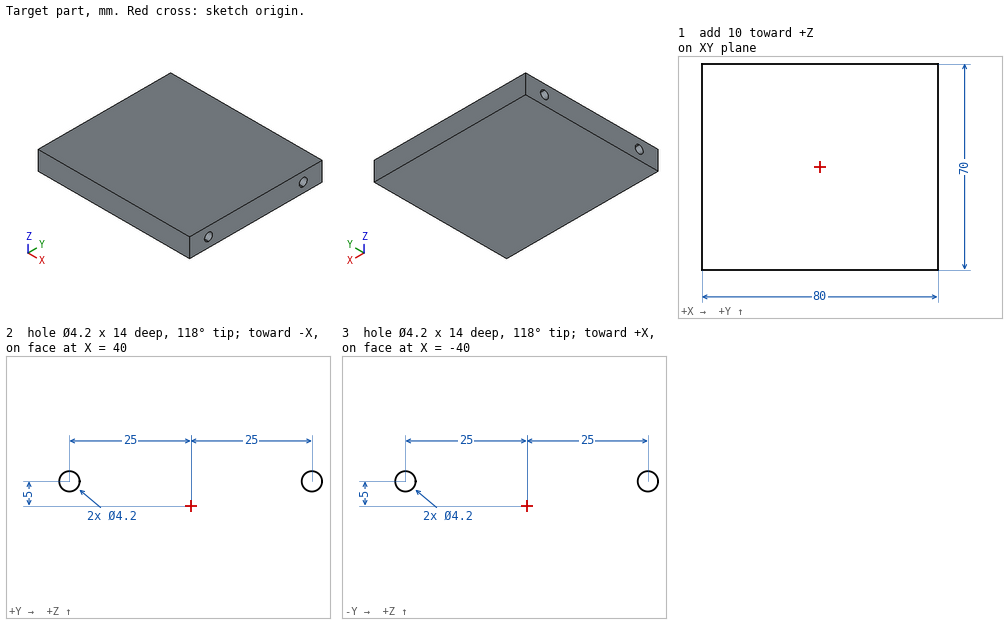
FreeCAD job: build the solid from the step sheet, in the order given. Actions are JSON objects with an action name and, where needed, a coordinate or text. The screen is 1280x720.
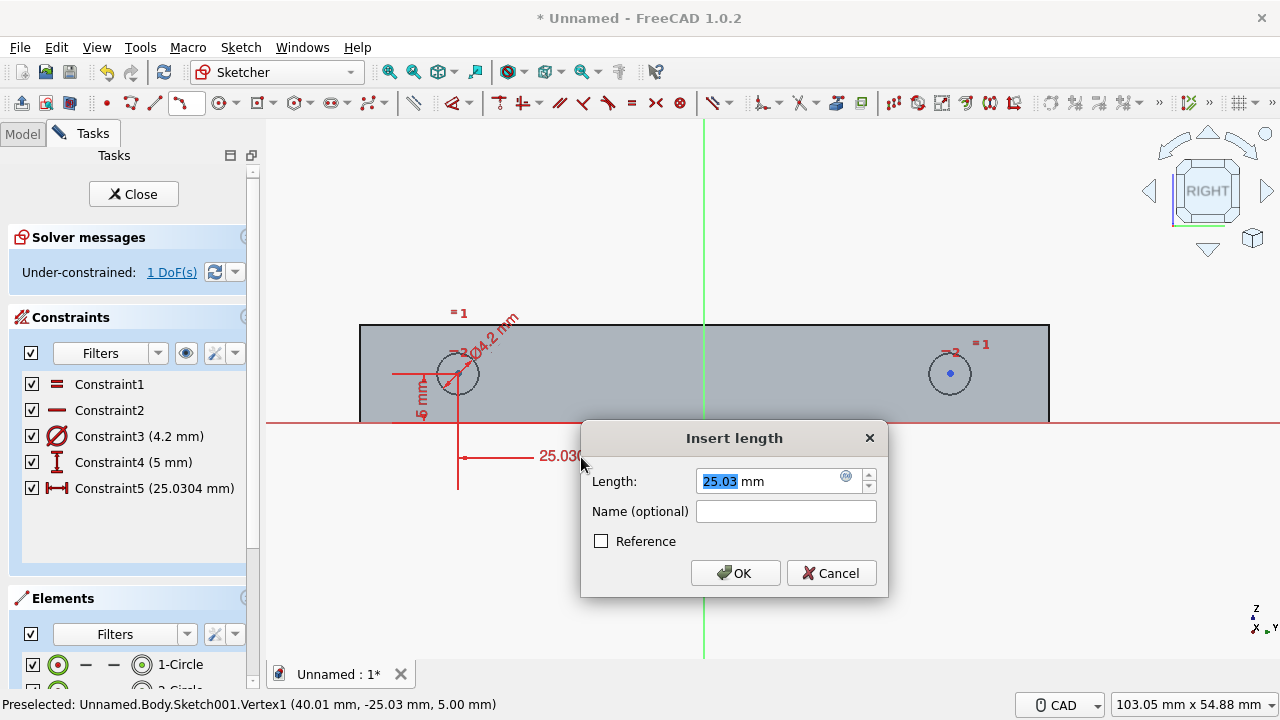
{"action": "type", "text": "25"}
{"action": "key", "text": "Return"}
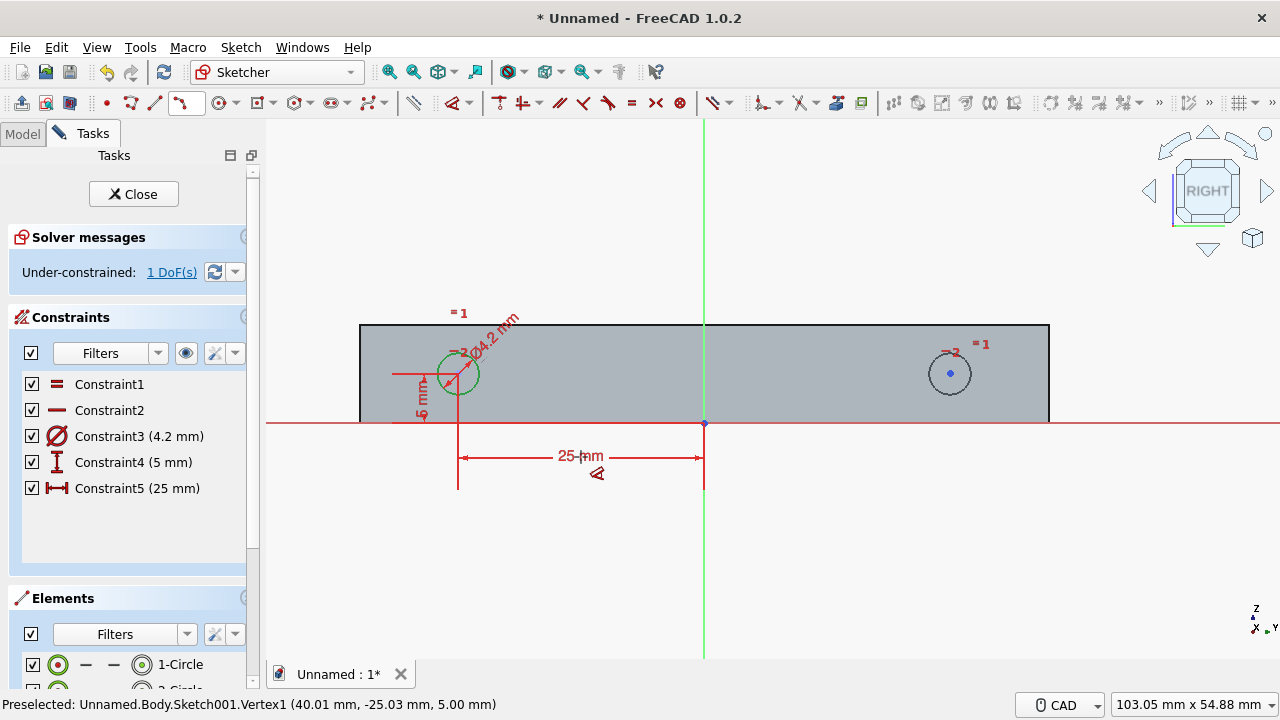
{"action": "left_click", "coordinate": [950, 374]}
{"action": "left_click", "coordinate": [827, 457]}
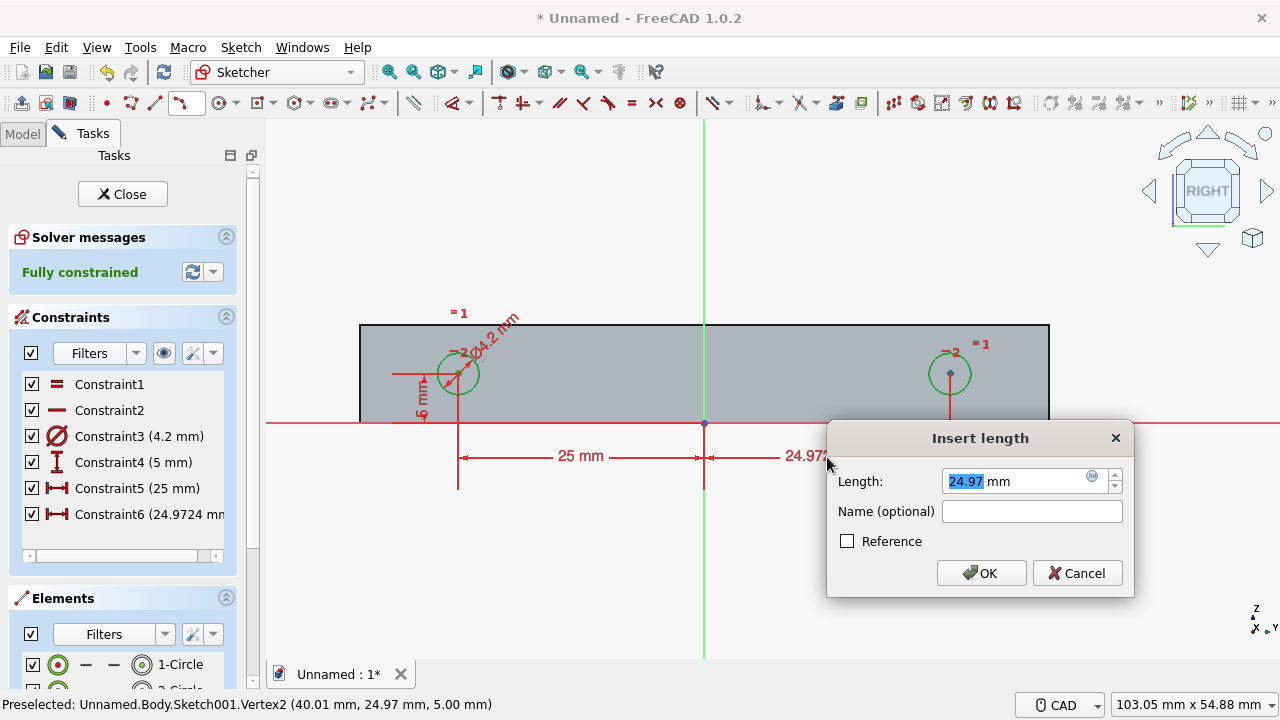
{"action": "type", "text": "25"}
{"action": "key", "text": "Return"}
{"action": "key", "text": "Escape"}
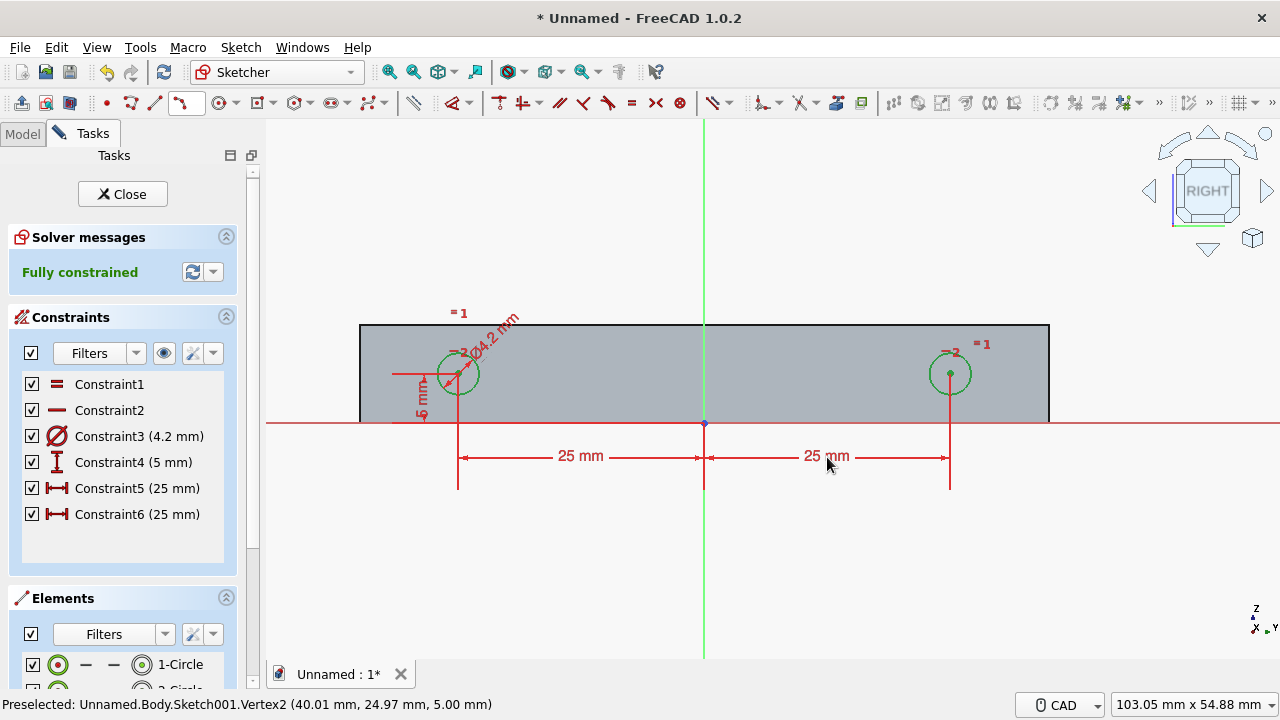
{"action": "left_click", "coordinate": [123, 194]}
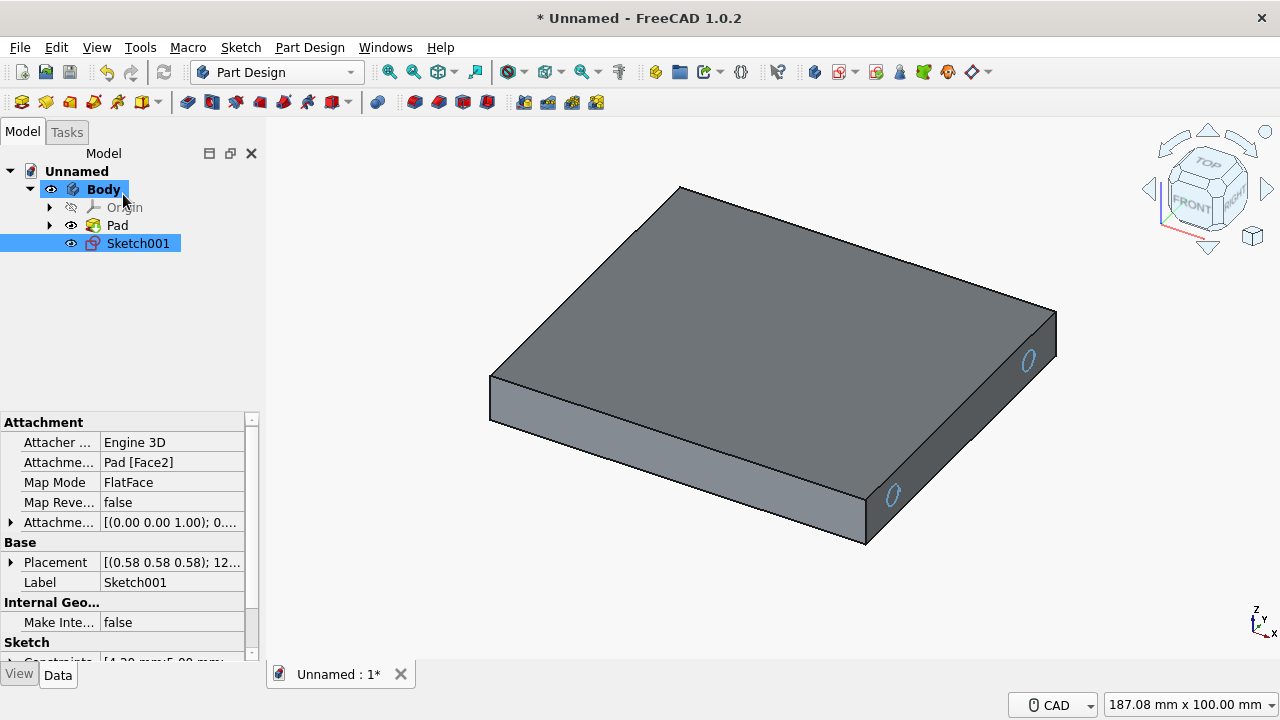
{"action": "left_click", "coordinate": [212, 102]}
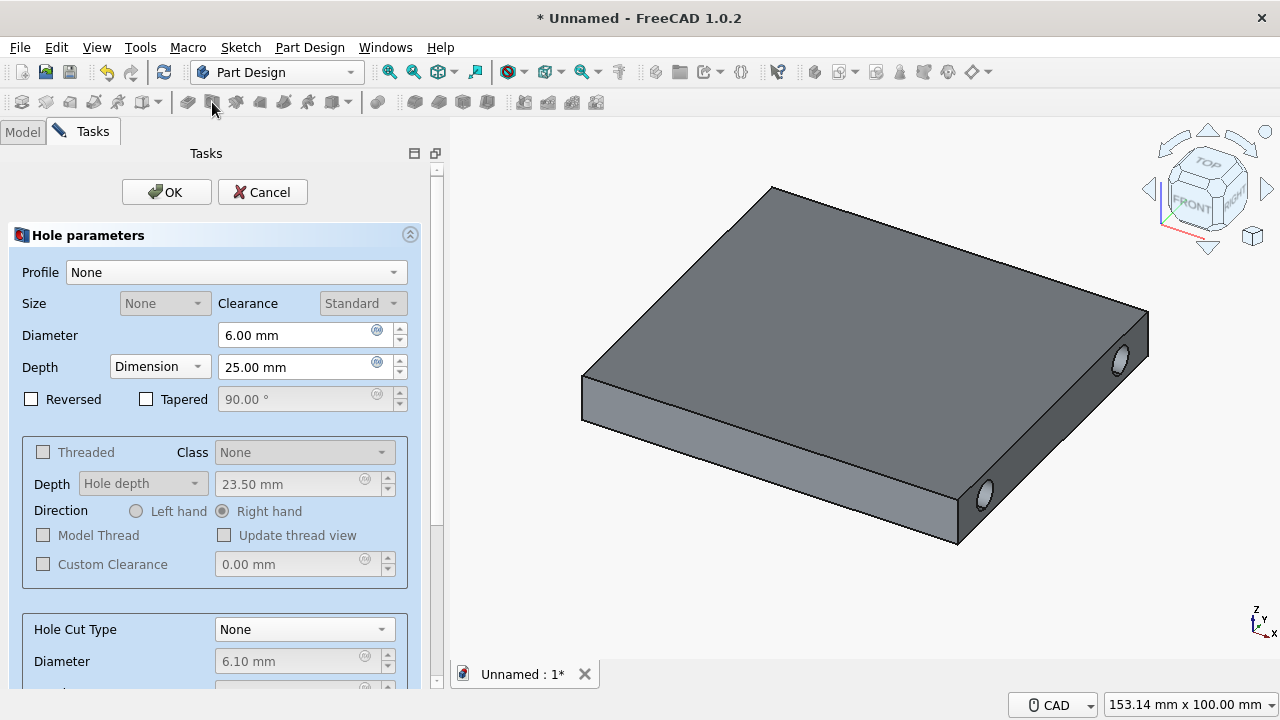
{"action": "triple_click", "coordinate": [305, 335]}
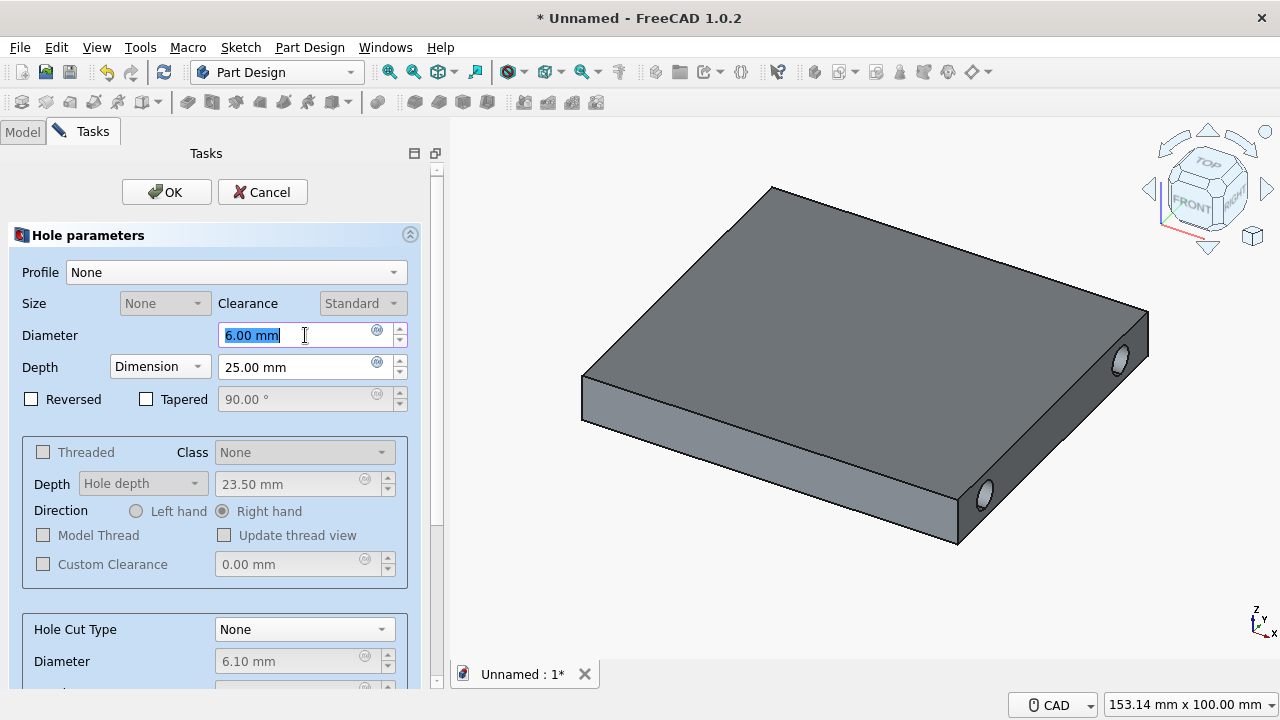
{"action": "type", "text": "4.2"}
{"action": "key", "text": "Tab"}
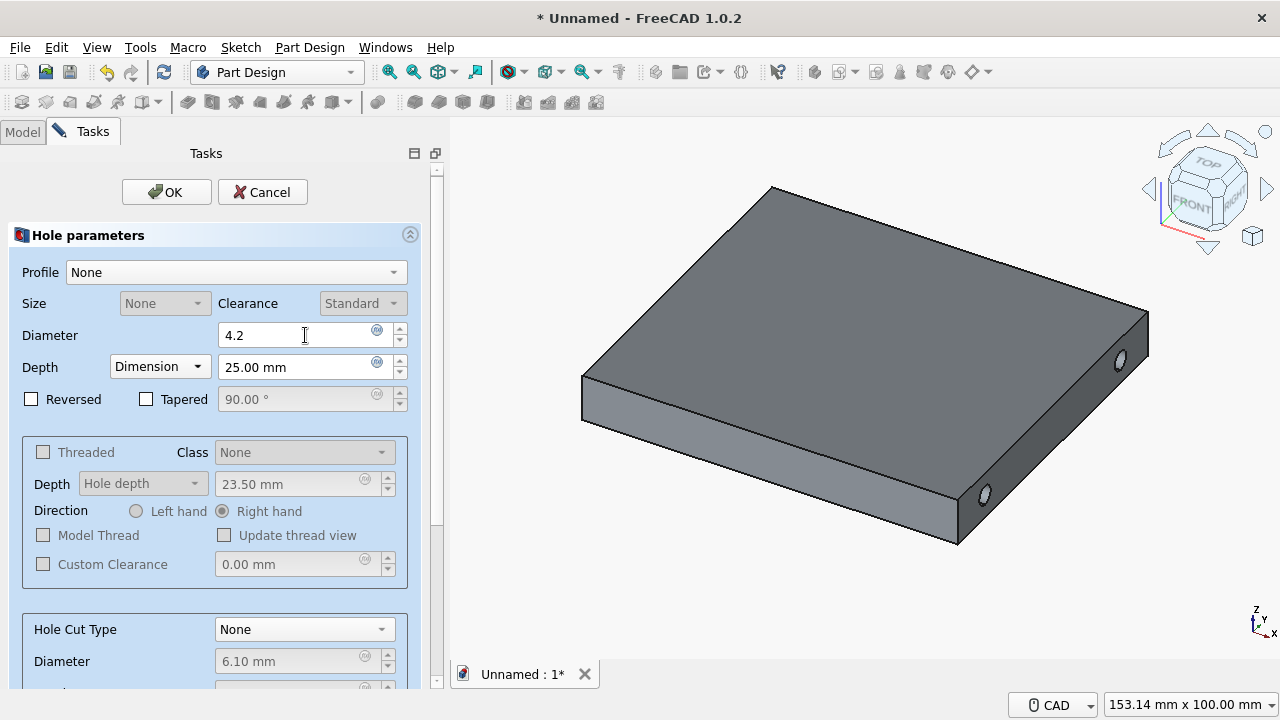
{"action": "triple_click", "coordinate": [305, 367]}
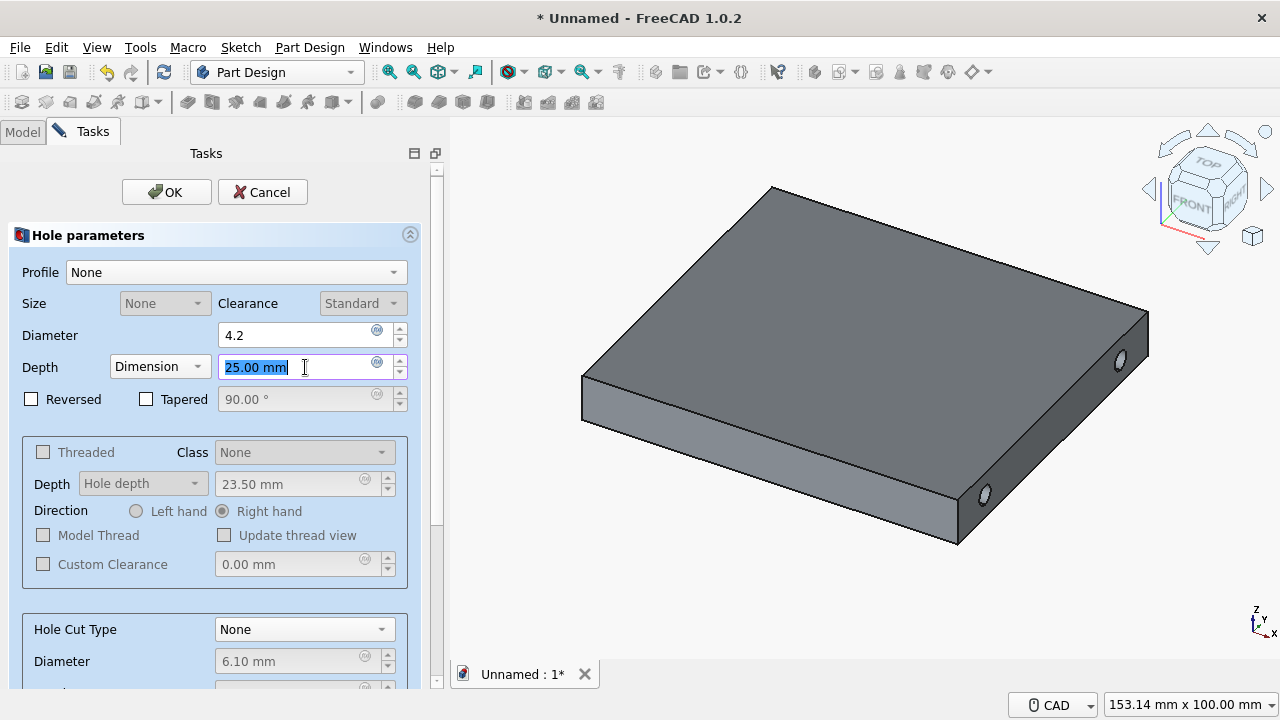
{"action": "type", "text": "14"}
{"action": "key", "text": "Tab"}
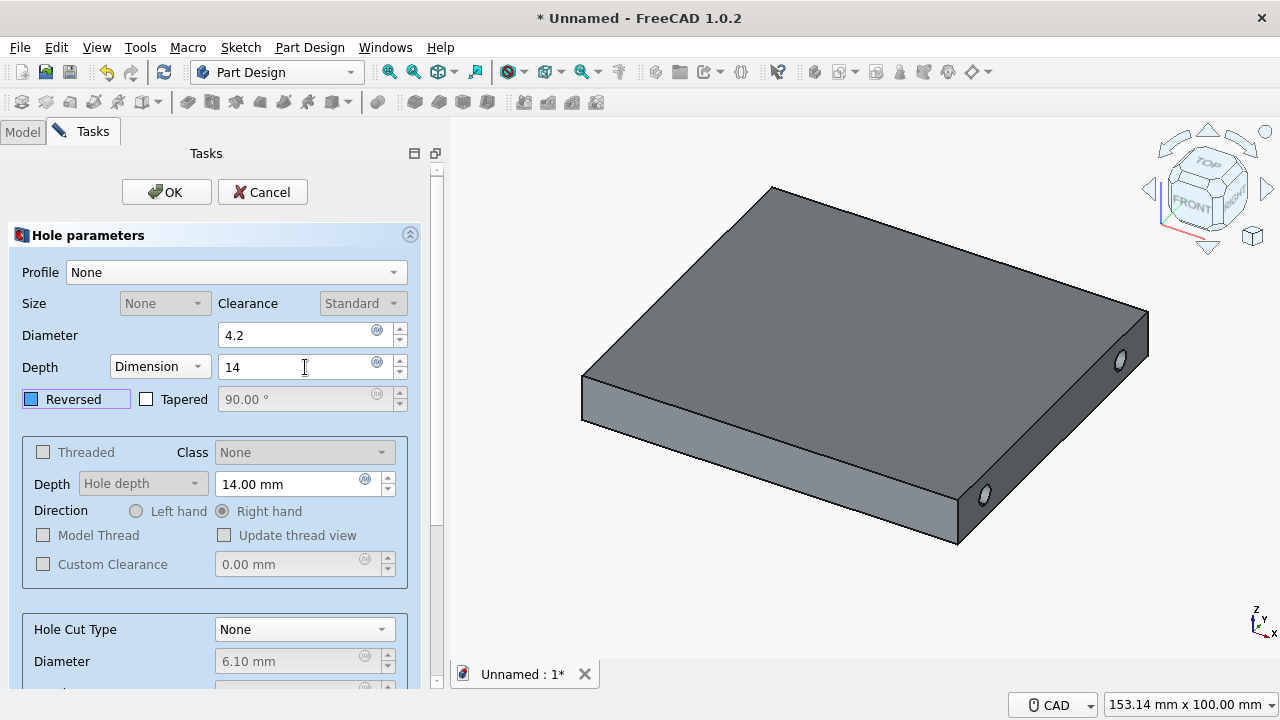
{"action": "left_click", "coordinate": [167, 192]}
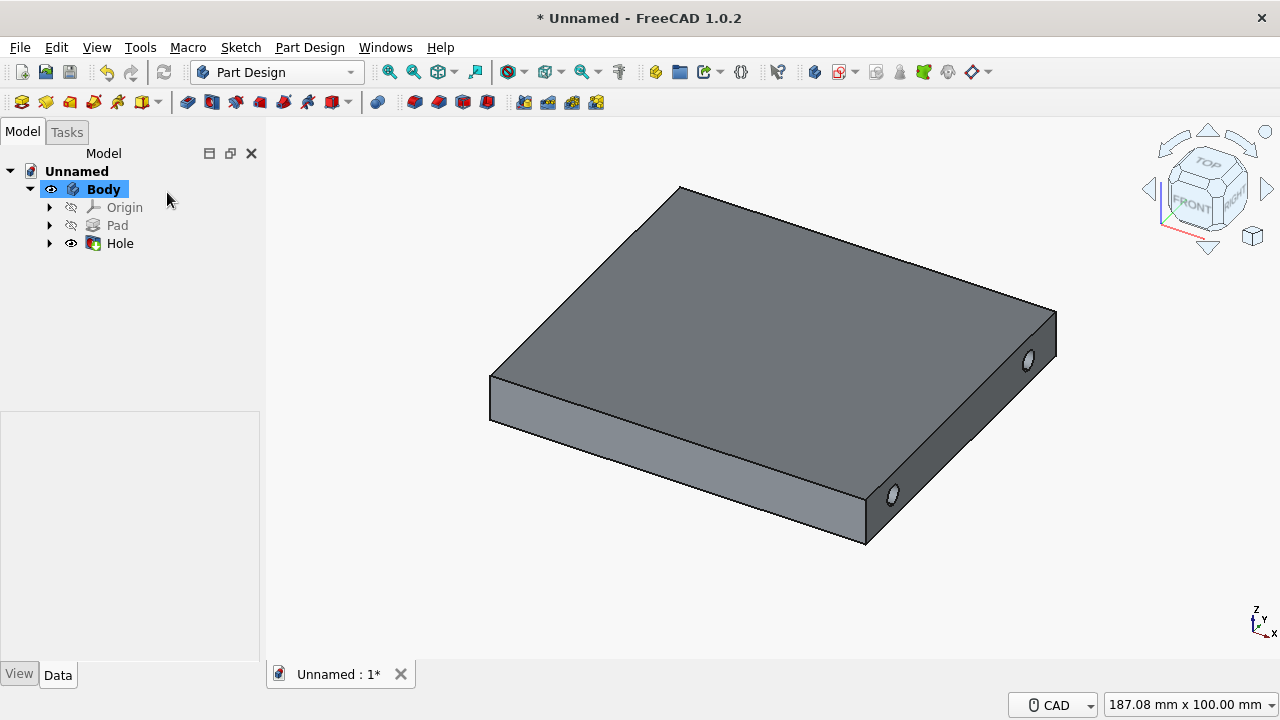
{"action": "key", "text": "6"}